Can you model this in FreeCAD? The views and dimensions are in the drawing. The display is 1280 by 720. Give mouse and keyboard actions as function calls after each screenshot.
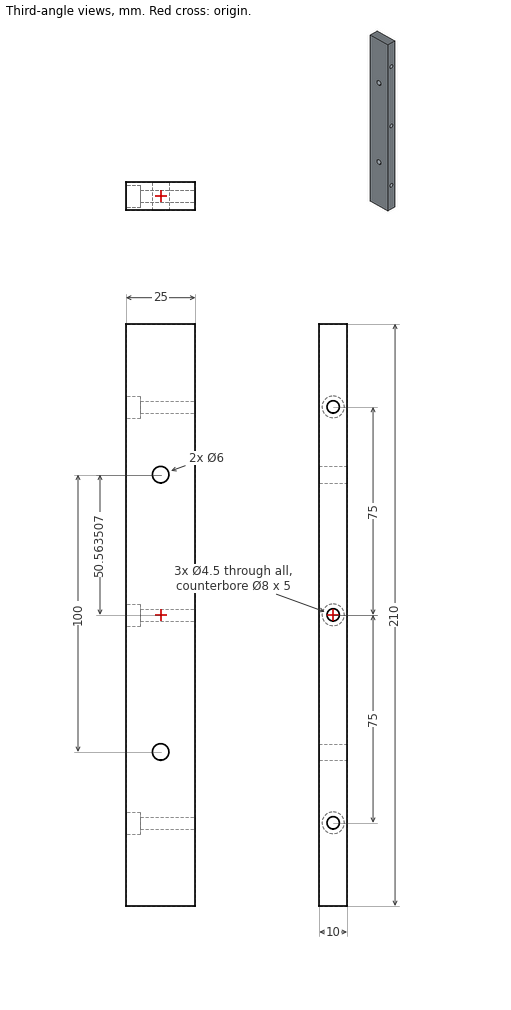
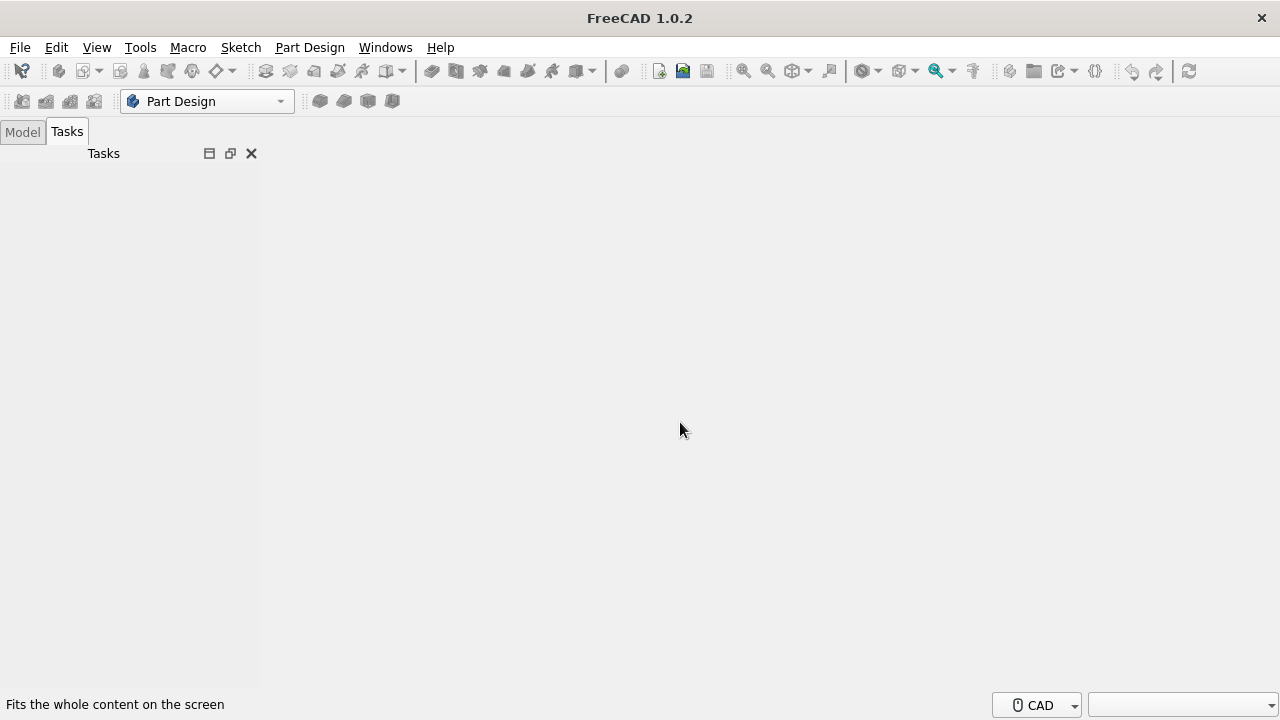
key(ctrl+n)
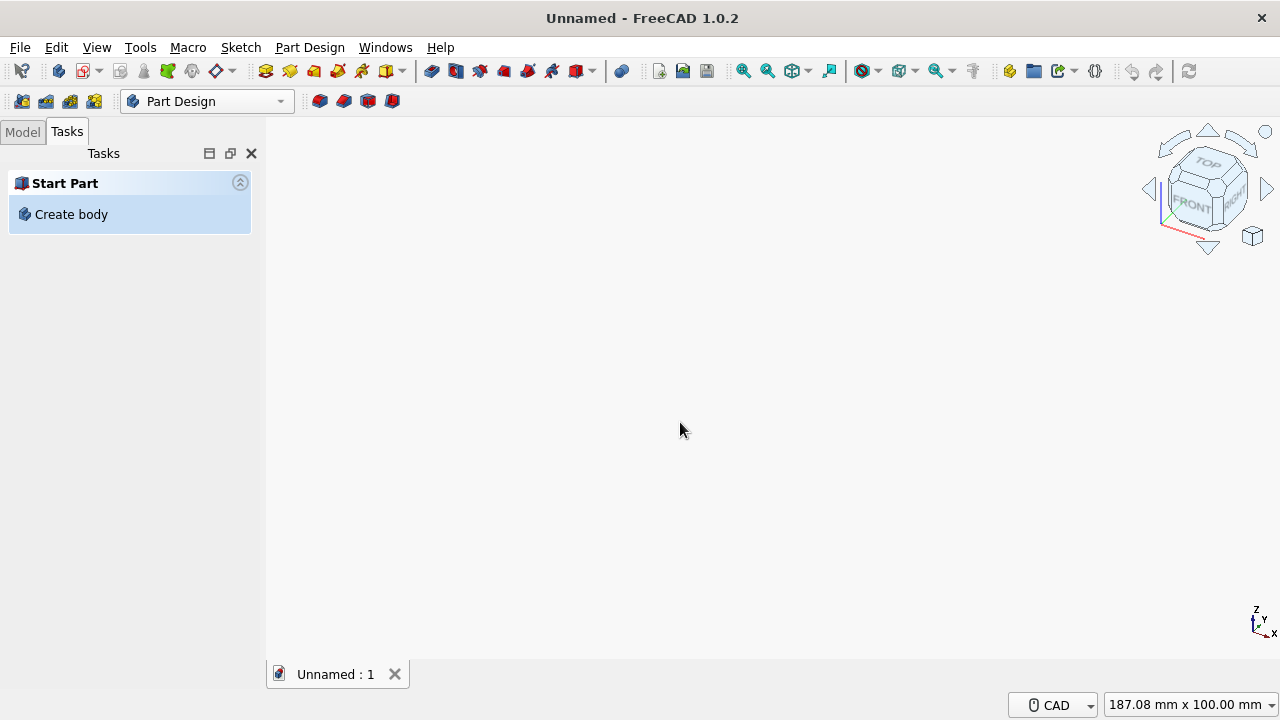
click(84, 72)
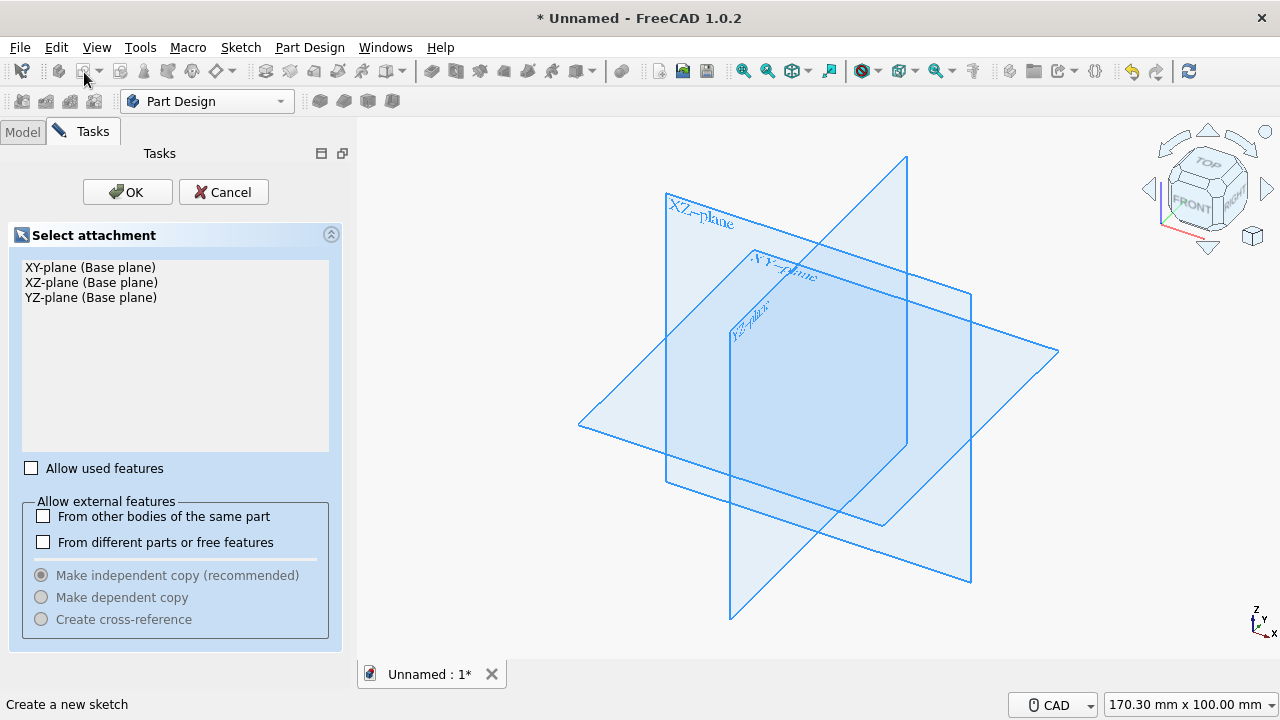
click(82, 298)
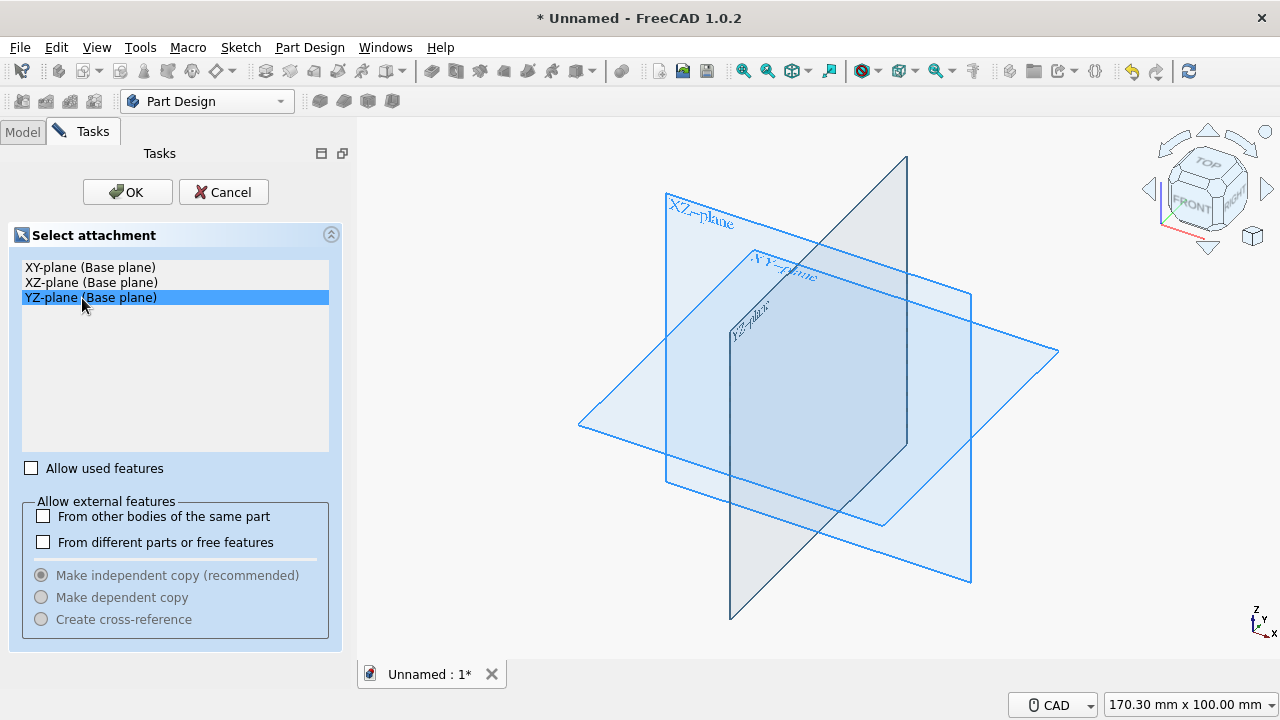
click(128, 192)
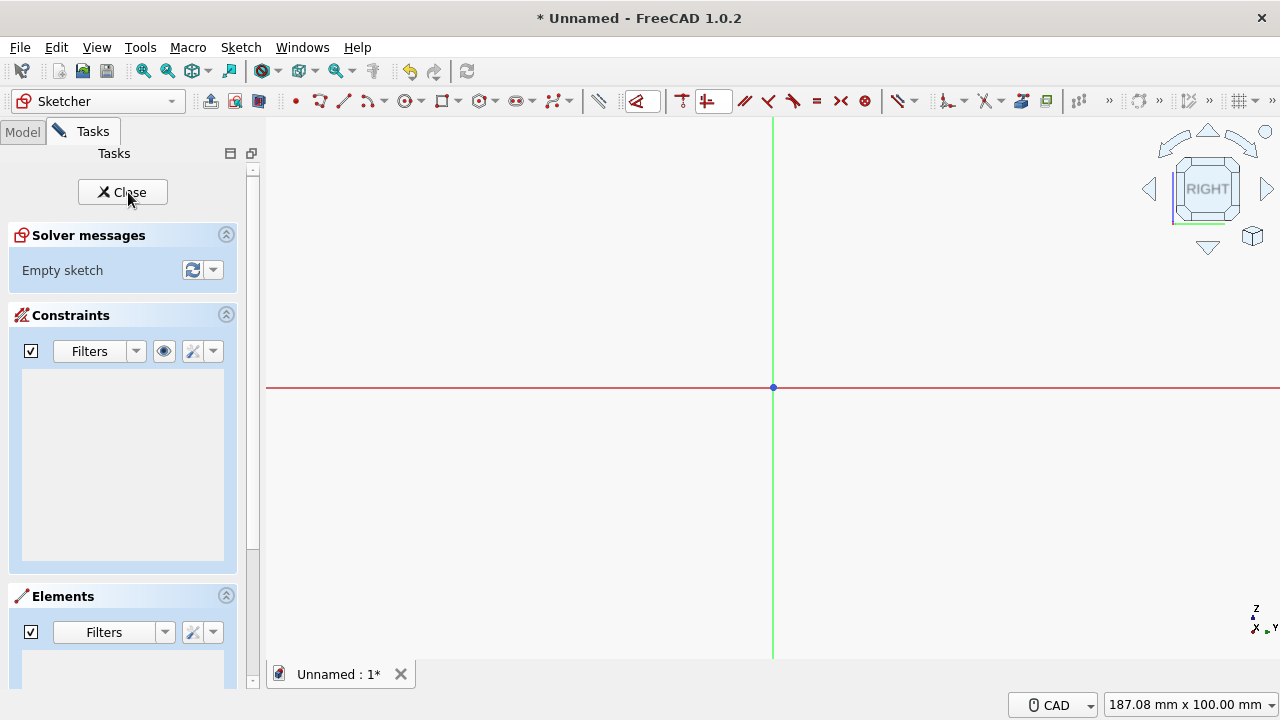
scroll(675, 388, down, 6)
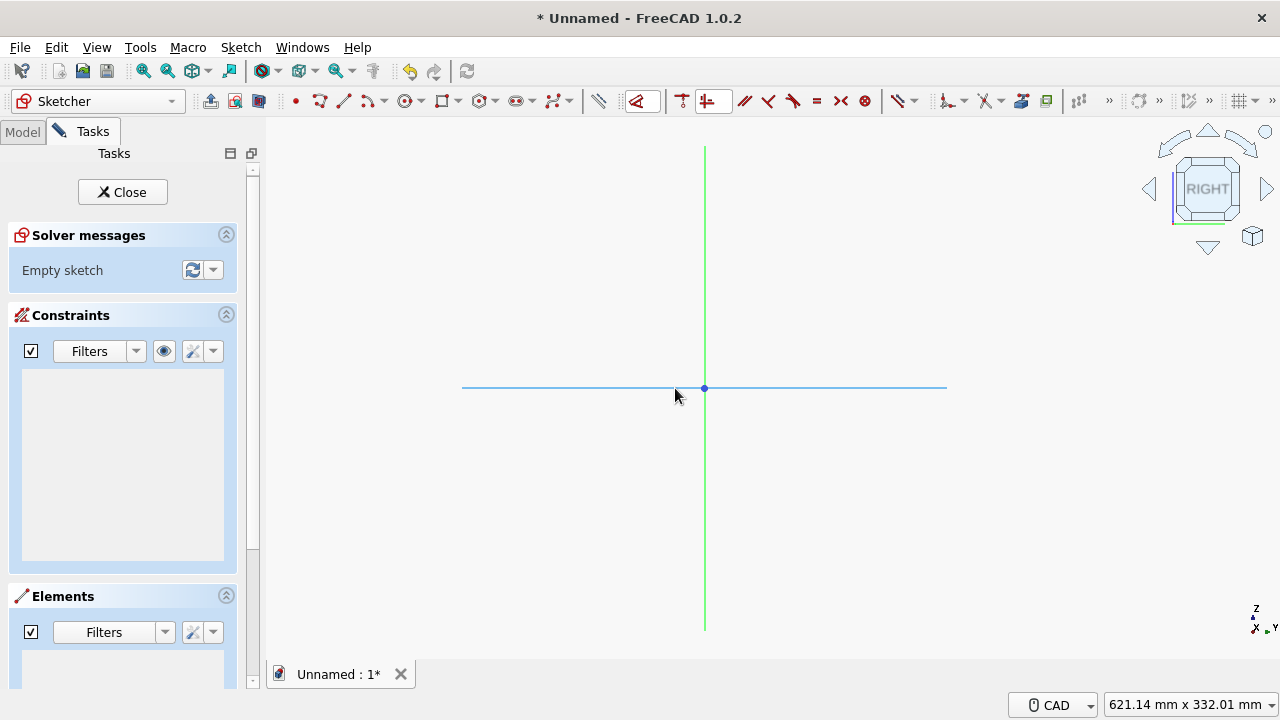
click(460, 102)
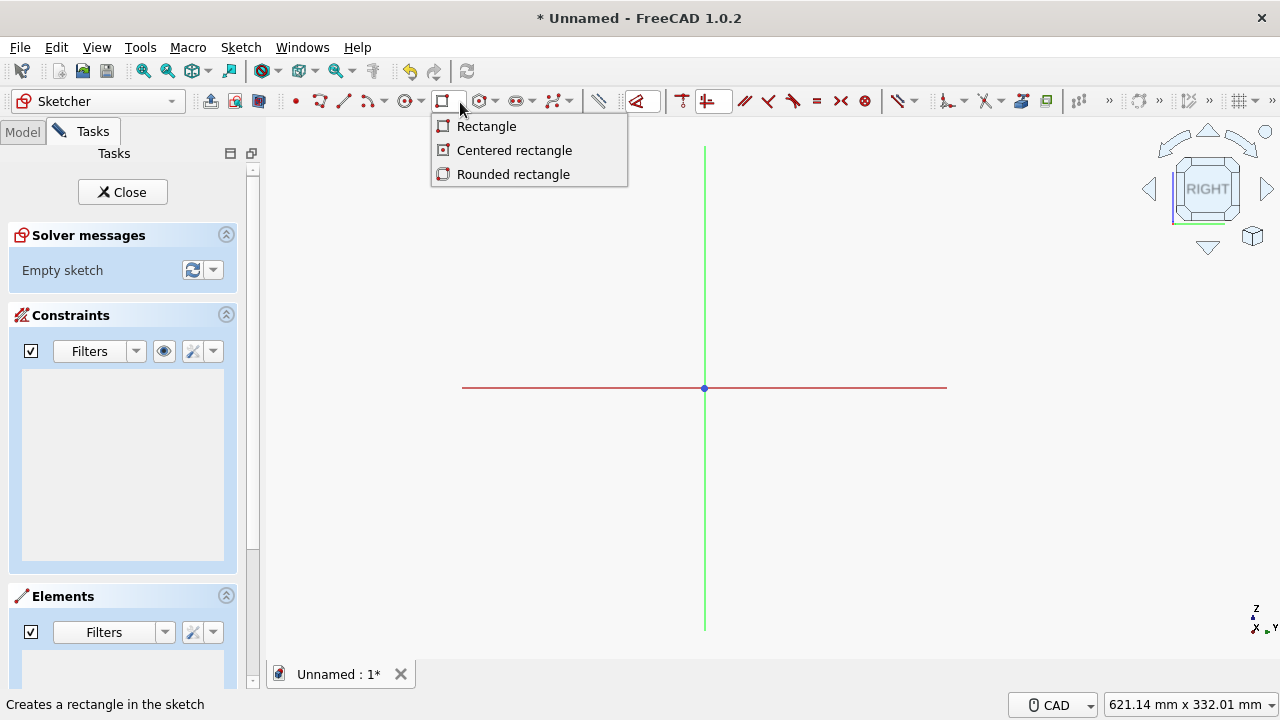
click(530, 150)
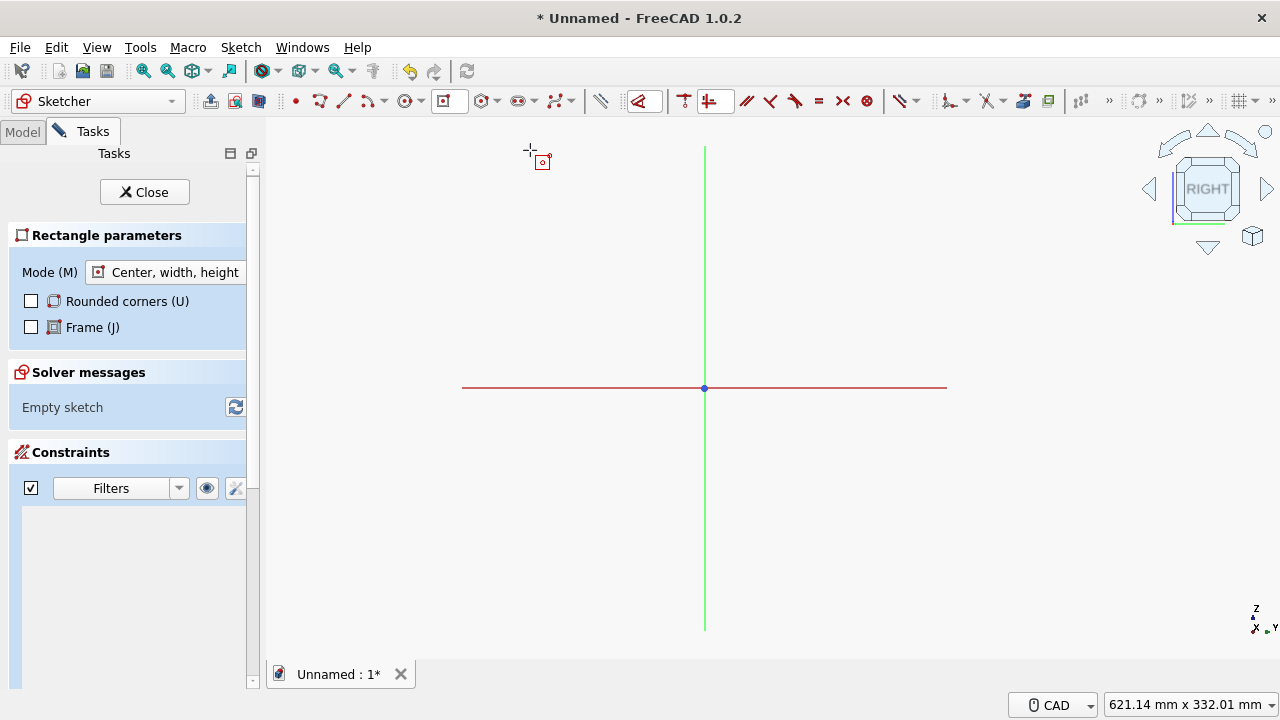
scroll(705, 388, up, 4)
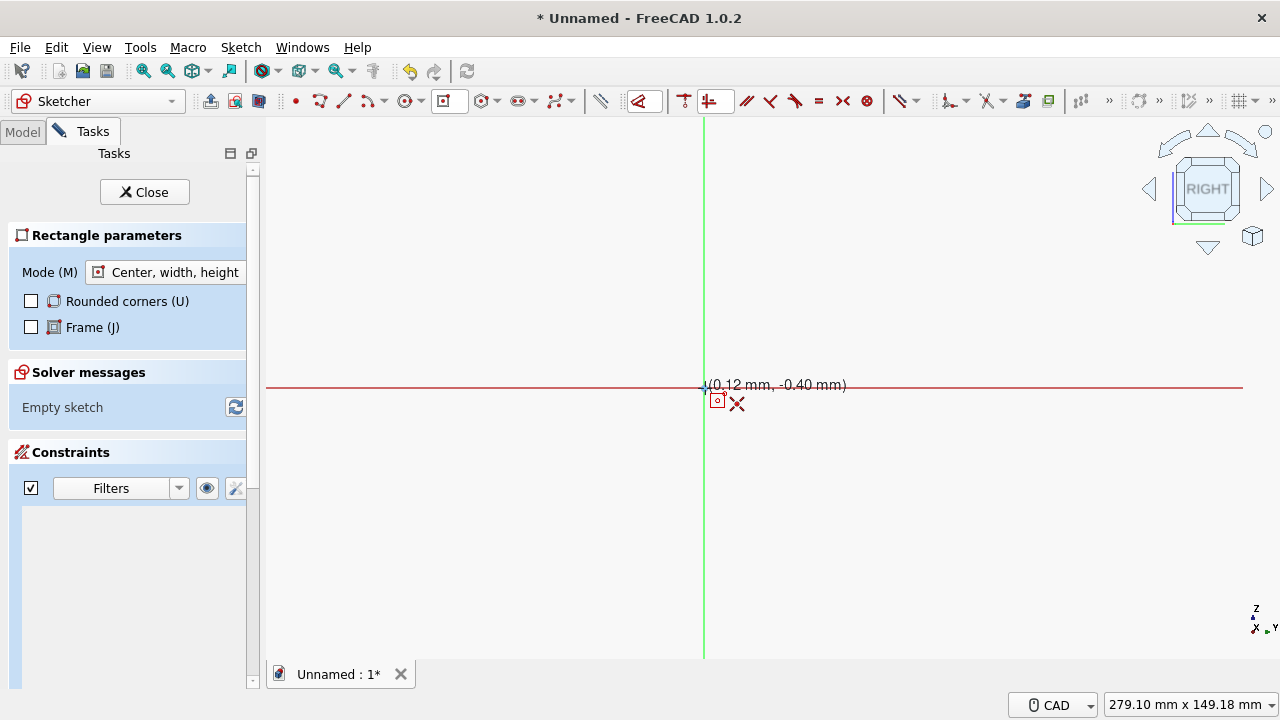
click(704, 388)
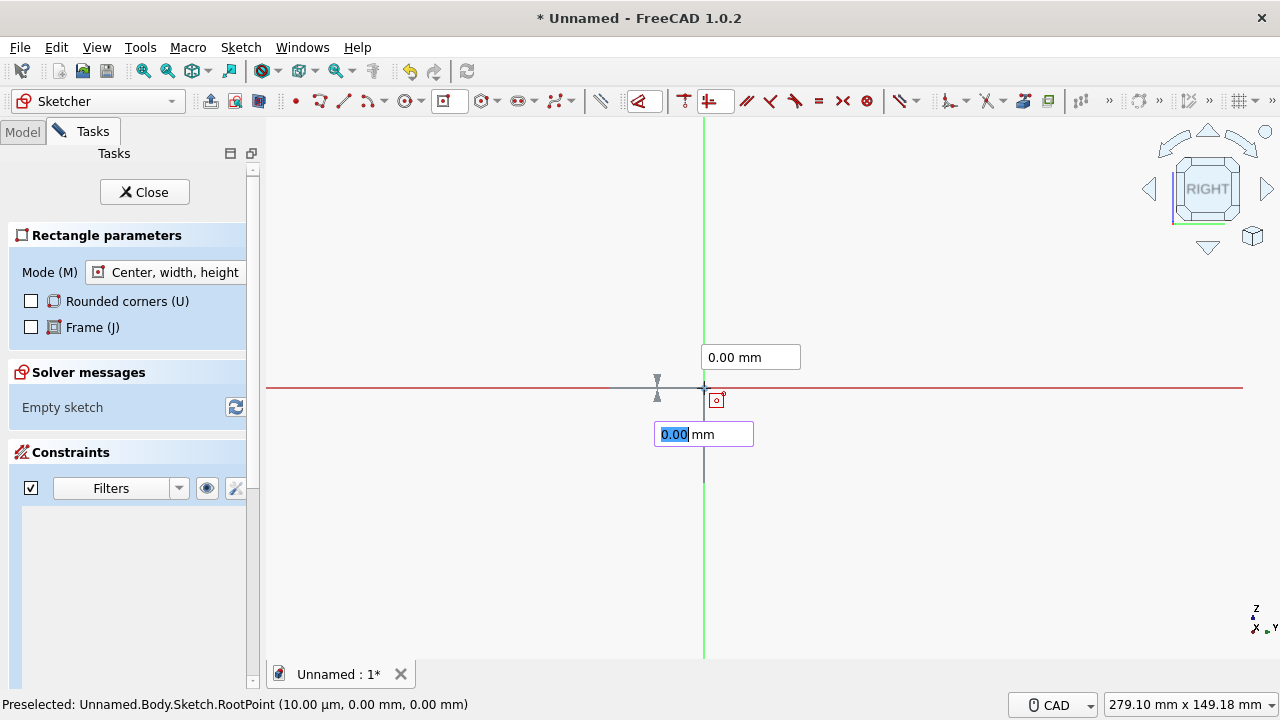
scroll(705, 388, down, 4)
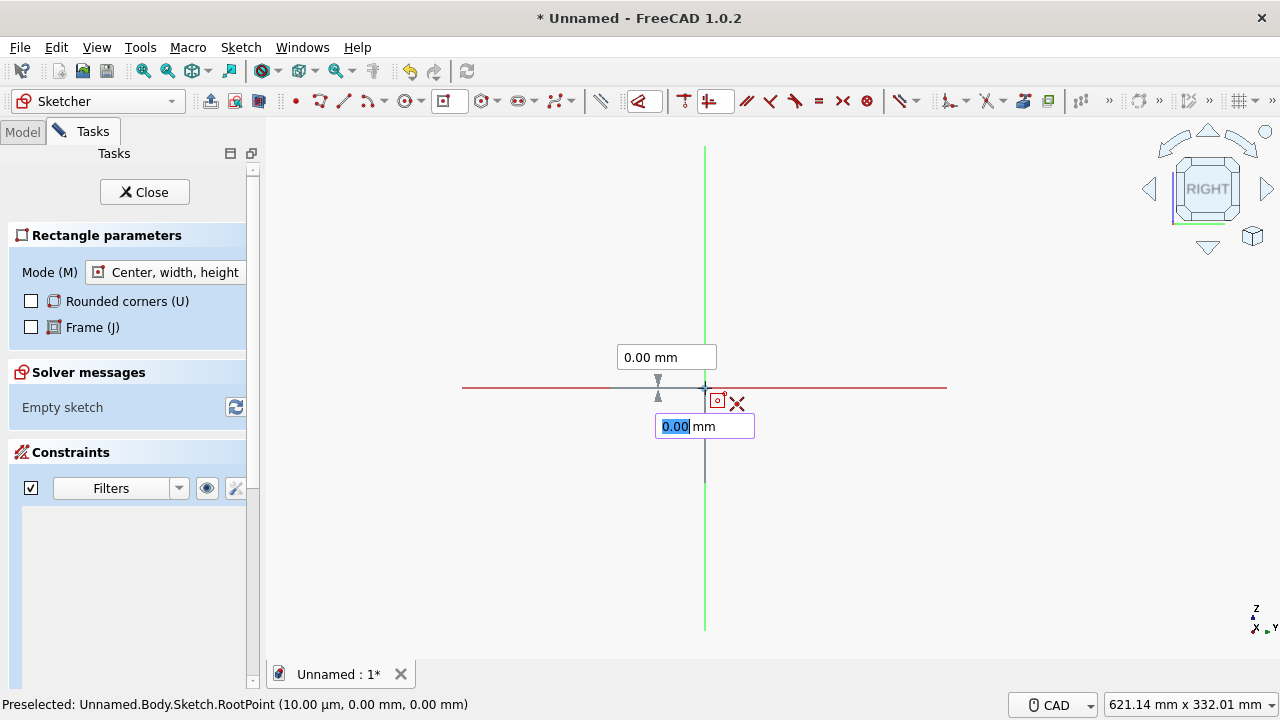
scroll(713, 217, up, 4)